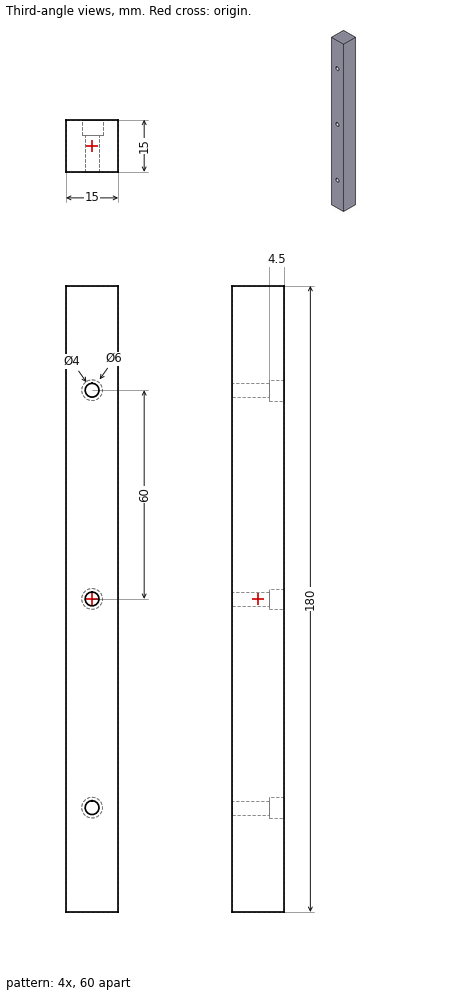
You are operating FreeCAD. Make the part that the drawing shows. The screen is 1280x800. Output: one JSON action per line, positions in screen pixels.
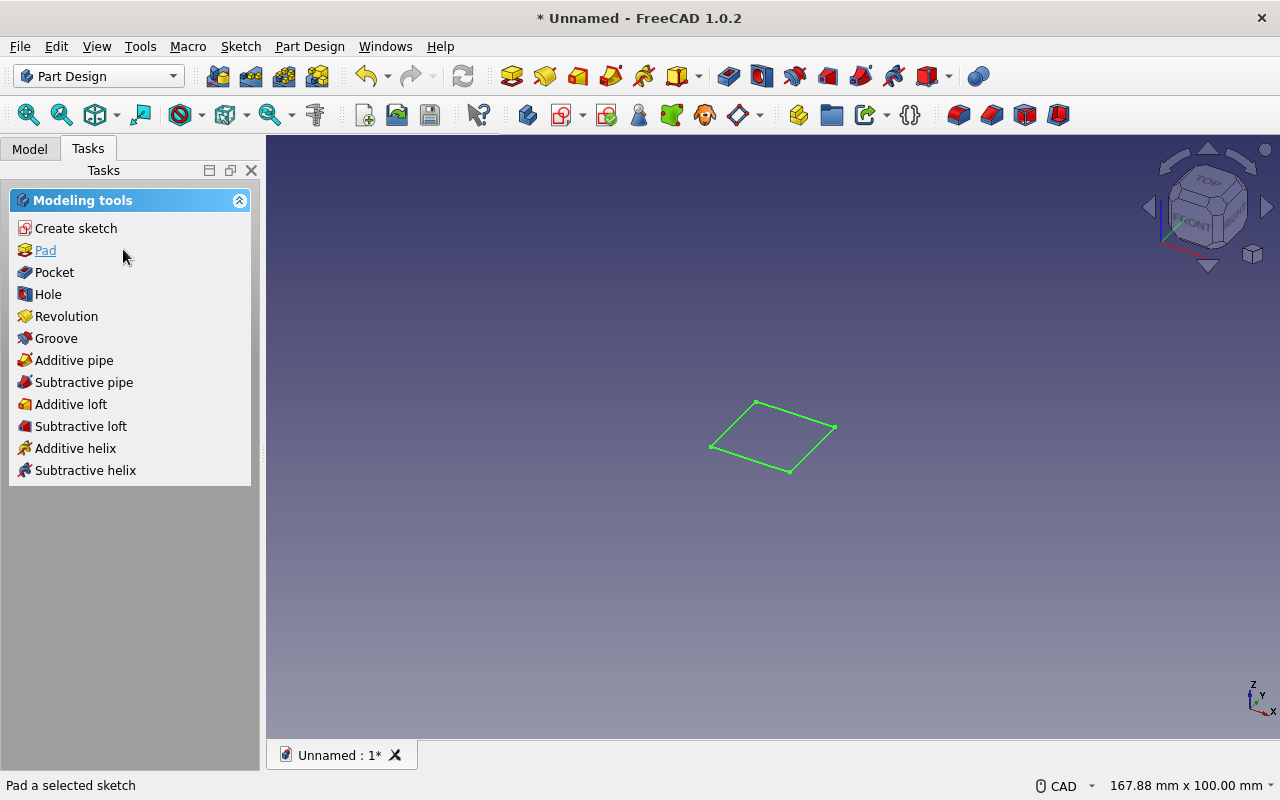
{"action": "left_click", "coordinate": [512, 76]}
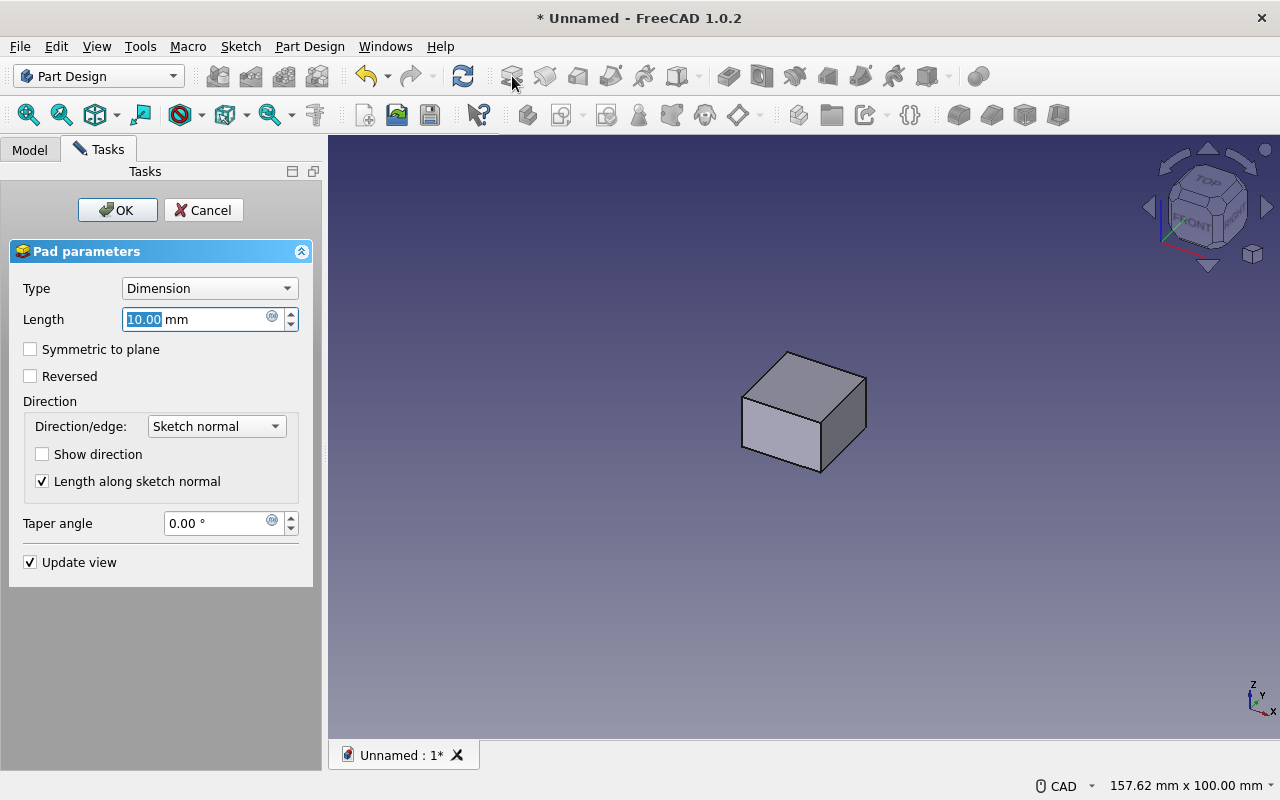
{"action": "type", "text": "180"}
{"action": "key", "text": "Tab"}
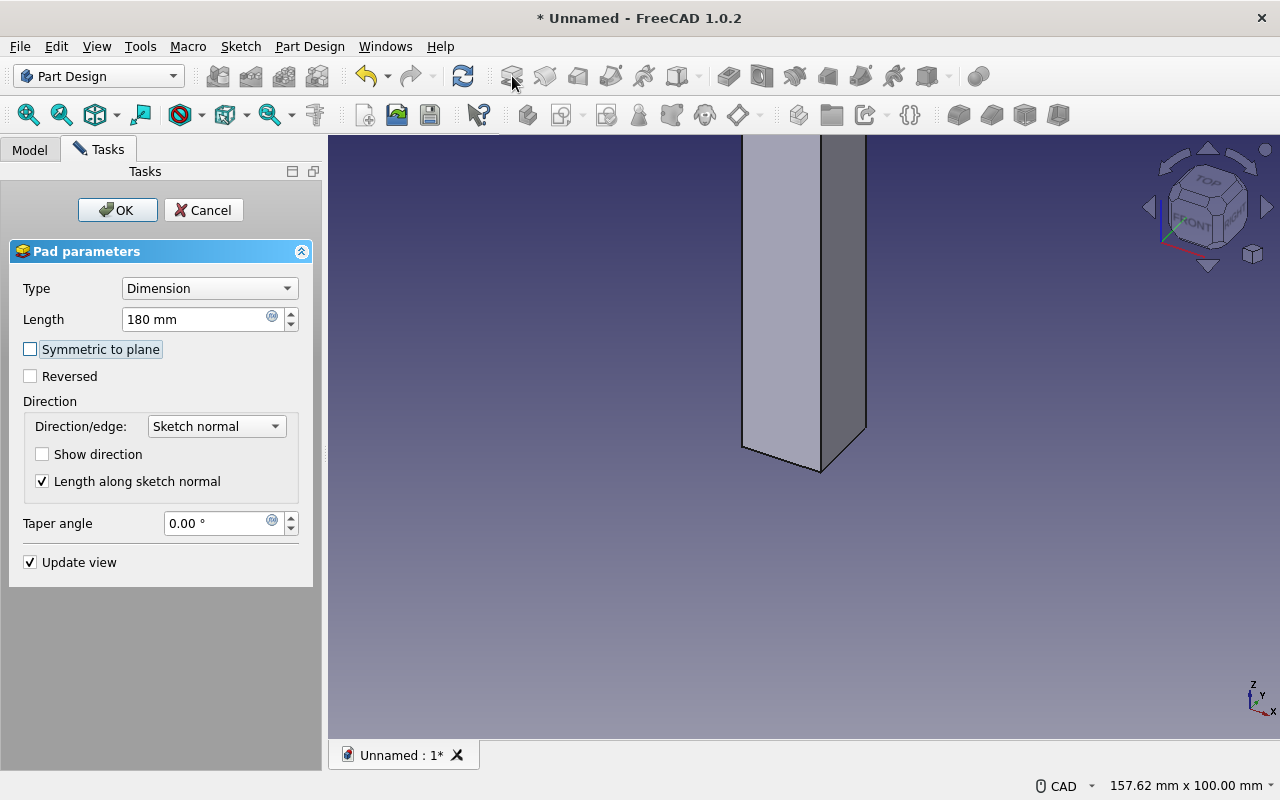
{"action": "left_click", "coordinate": [31, 349]}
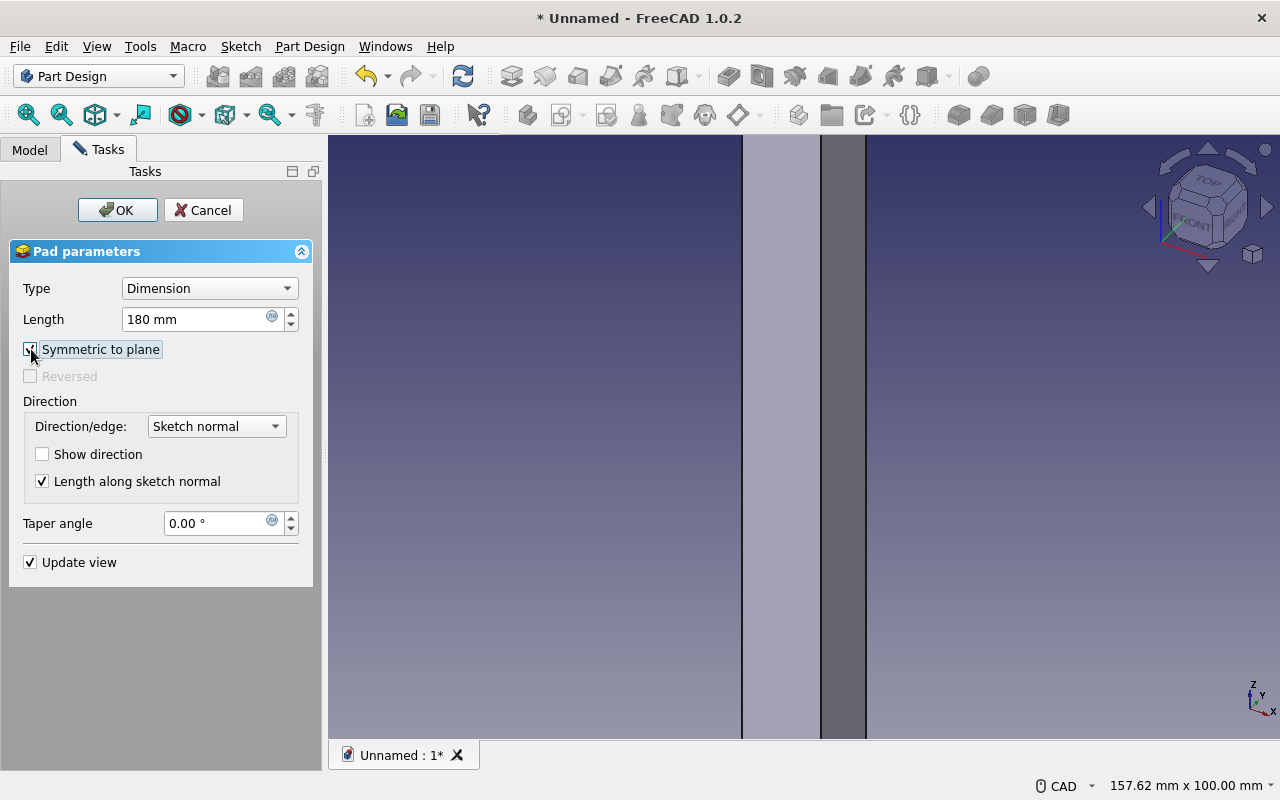
{"action": "left_click", "coordinate": [118, 210]}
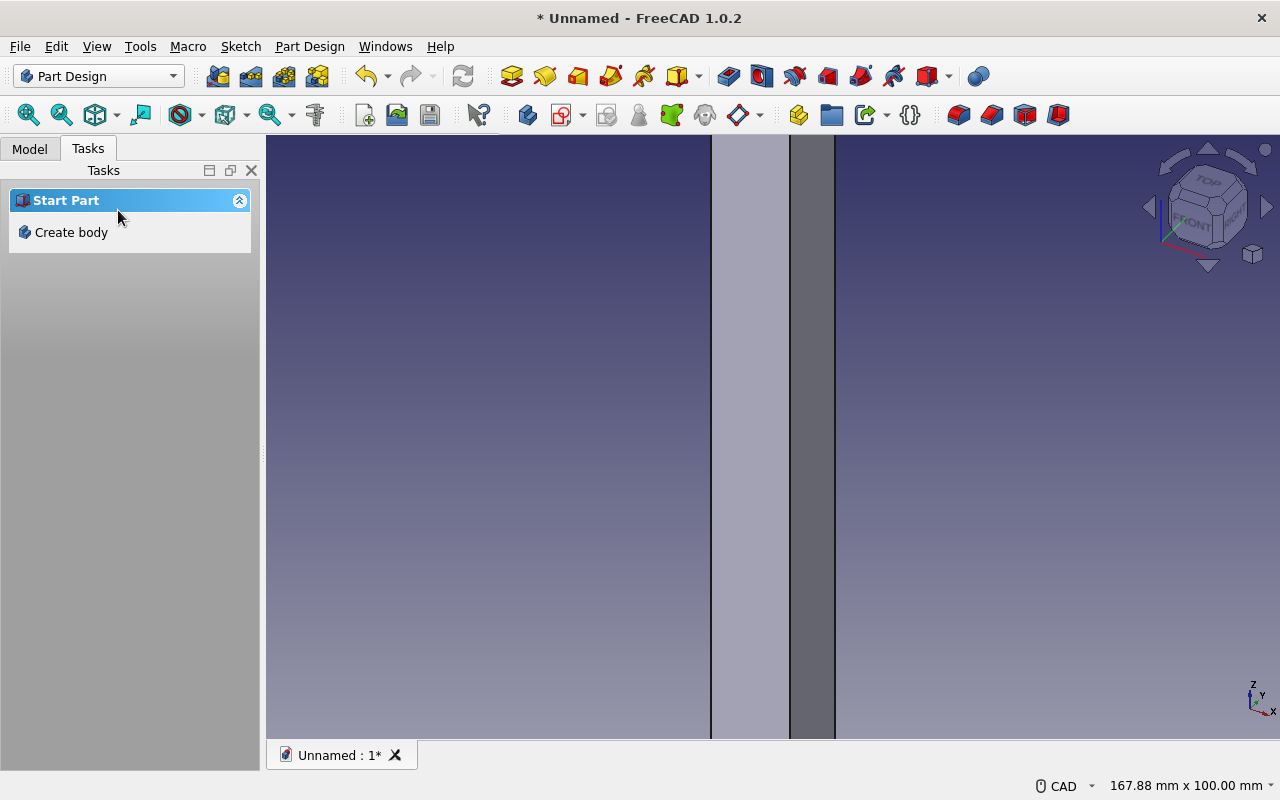
{"action": "left_click", "coordinate": [29, 116]}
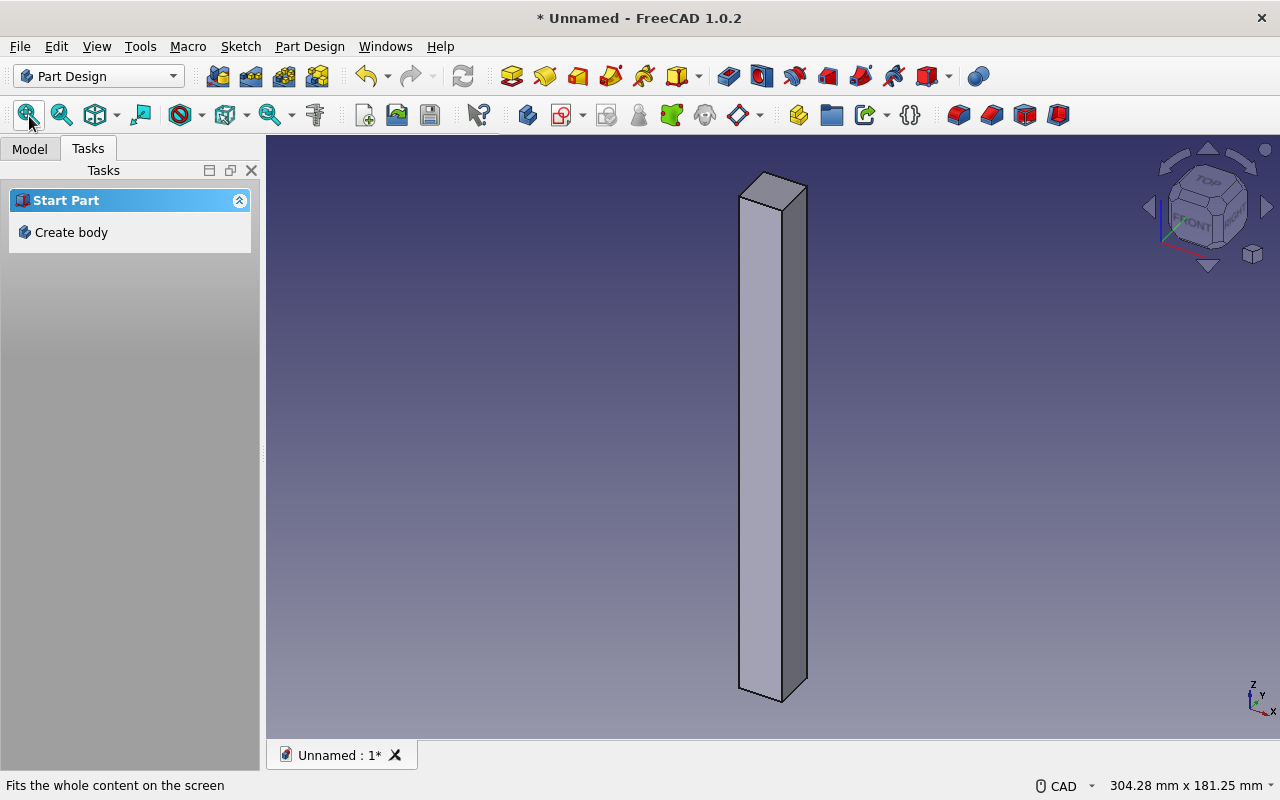
{"action": "key", "text": "4"}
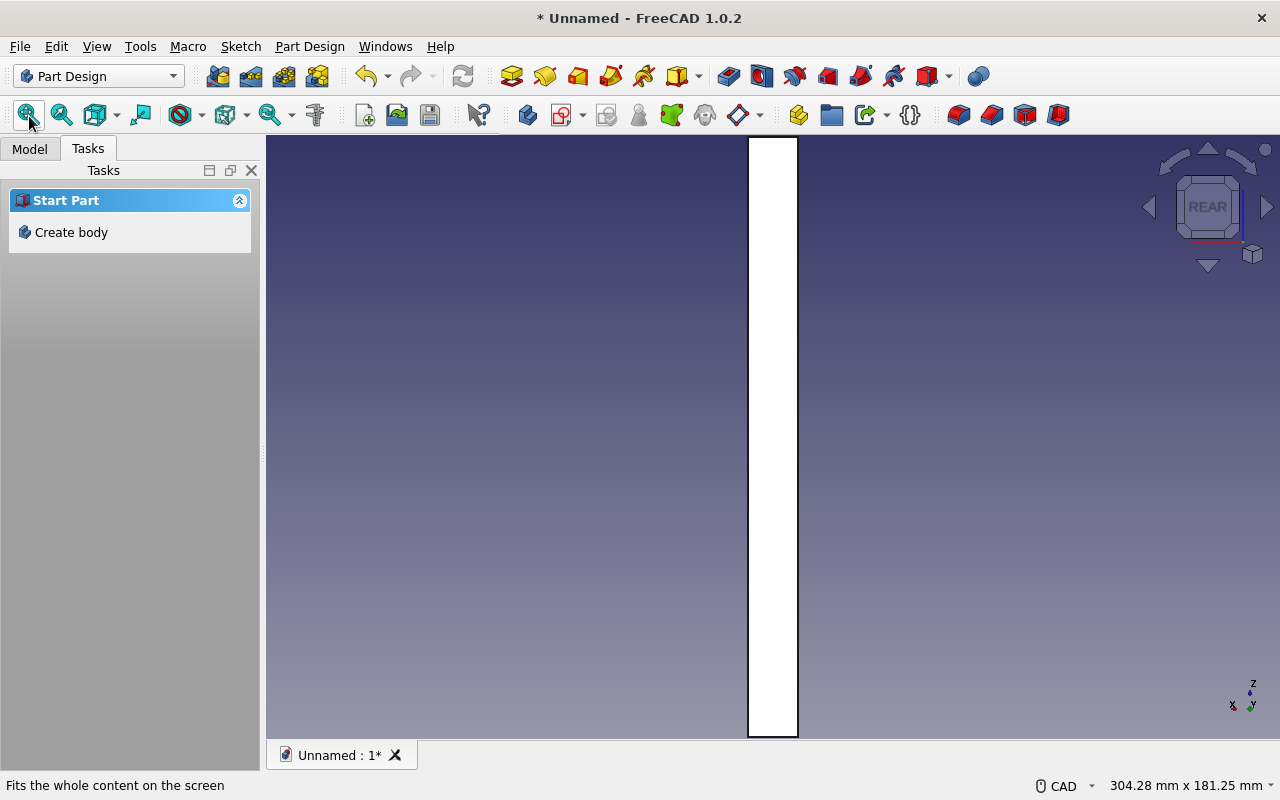
{"action": "left_click", "coordinate": [773, 179]}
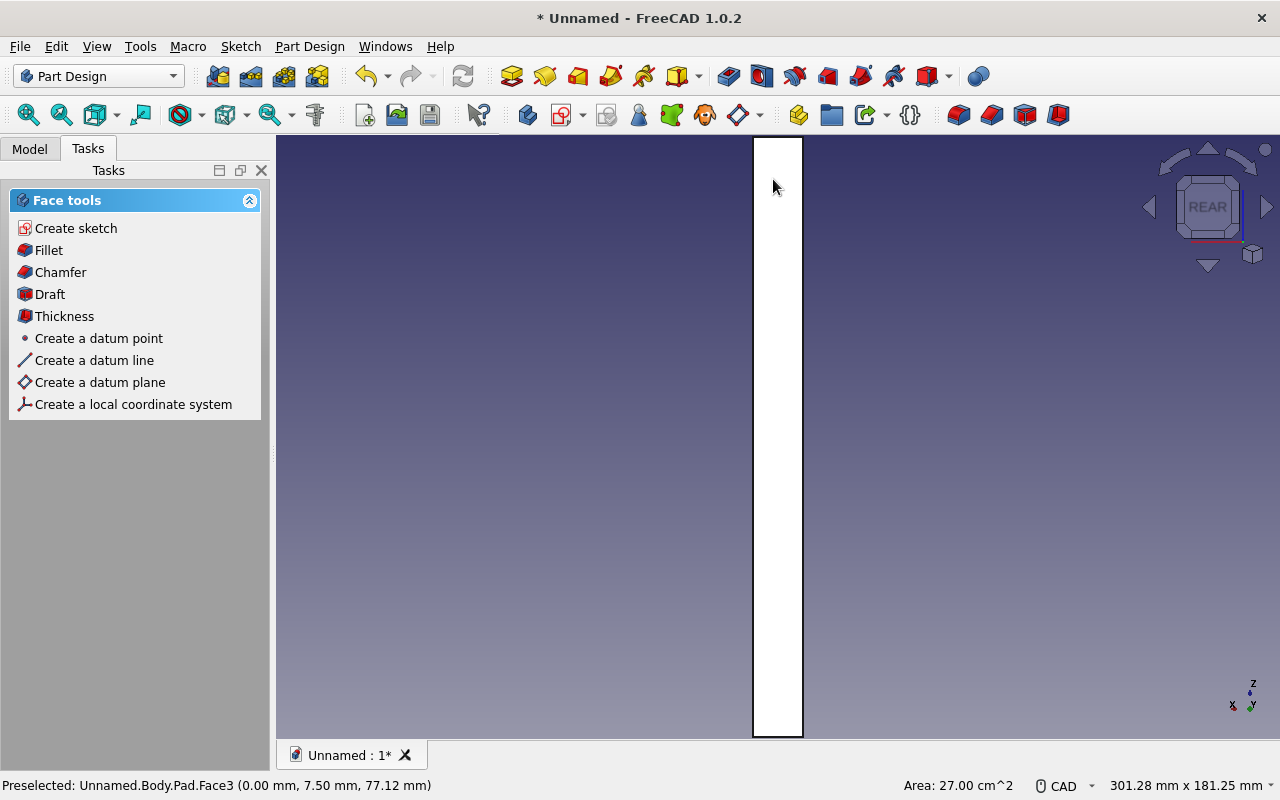
{"action": "left_click", "coordinate": [560, 116]}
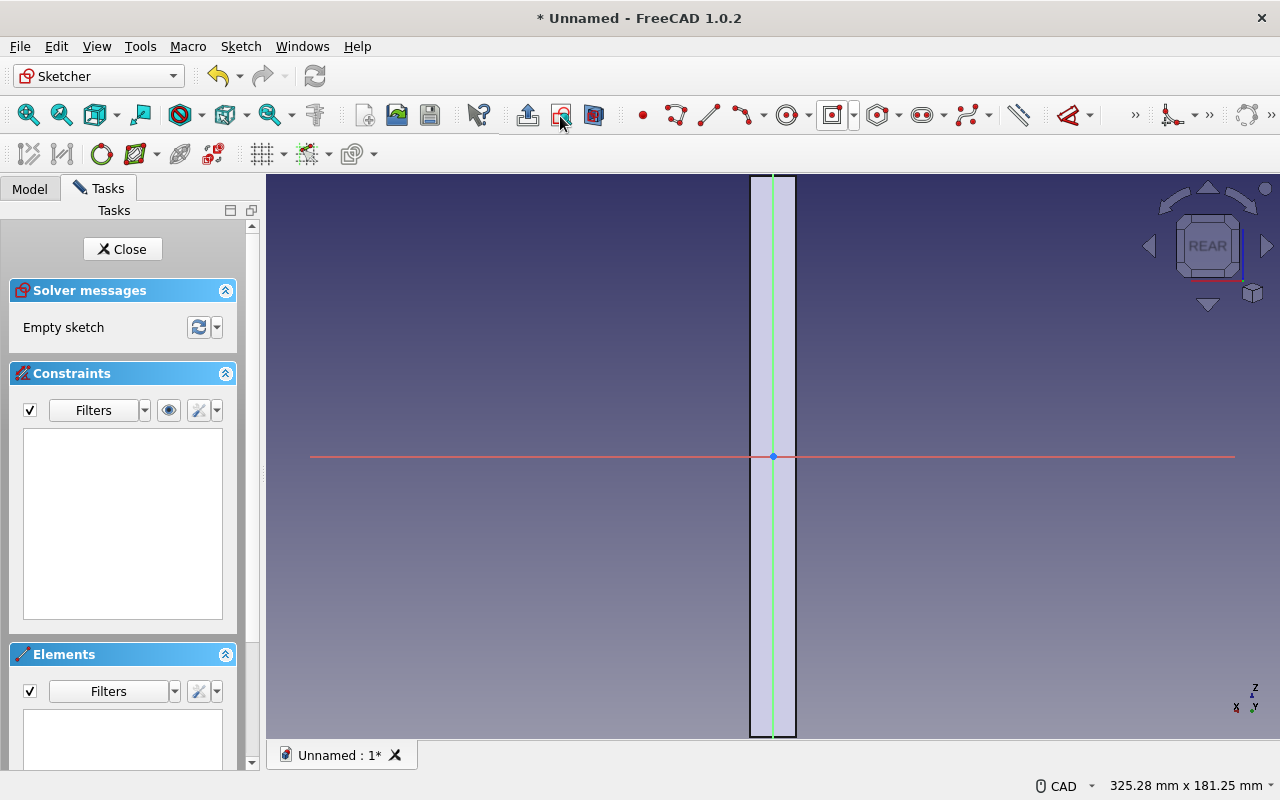
{"action": "scroll", "coordinate": [777, 260], "scroll_direction": "up", "scroll_amount": 15}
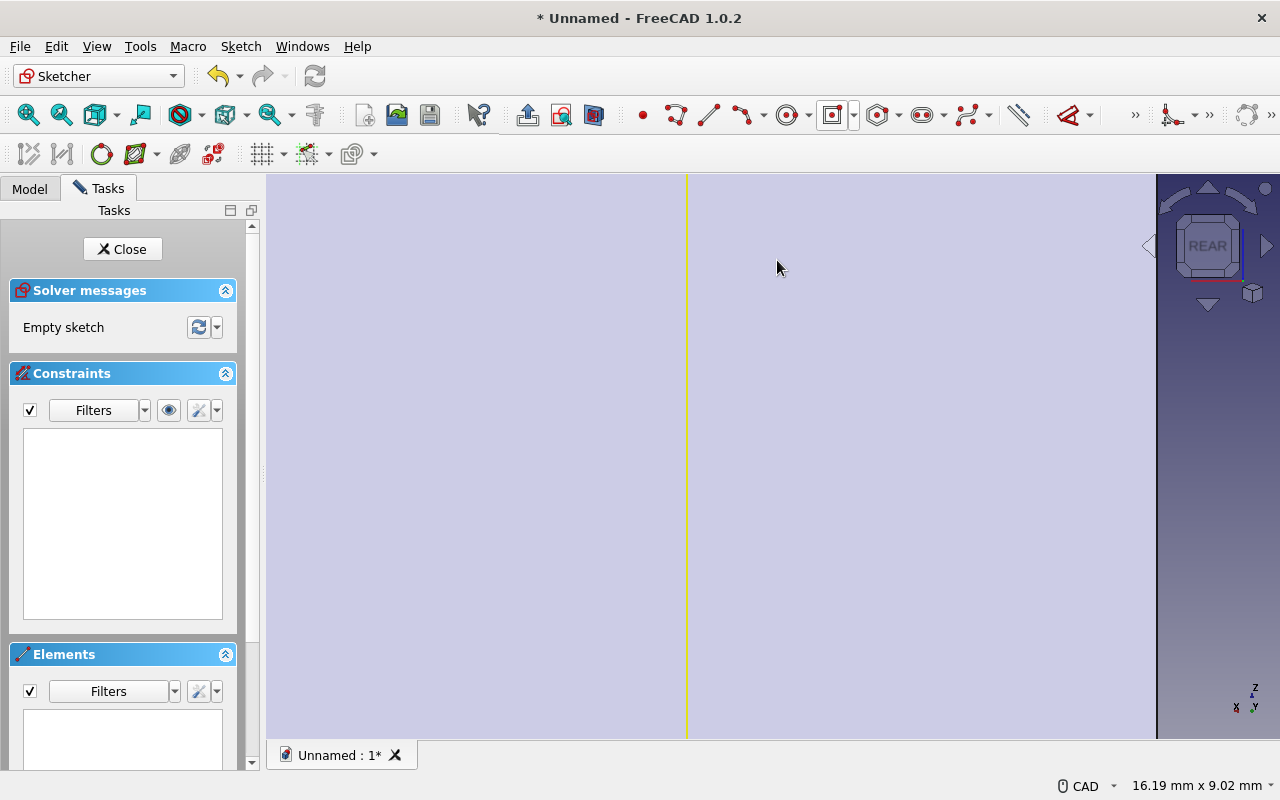
{"action": "key", "text": "g c"}